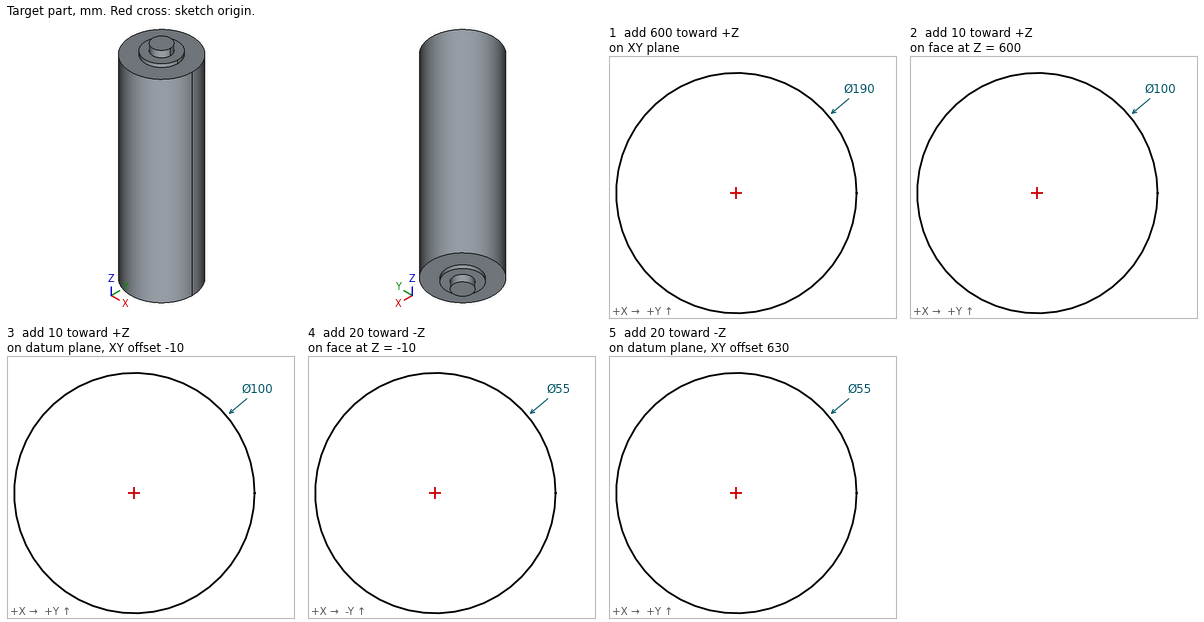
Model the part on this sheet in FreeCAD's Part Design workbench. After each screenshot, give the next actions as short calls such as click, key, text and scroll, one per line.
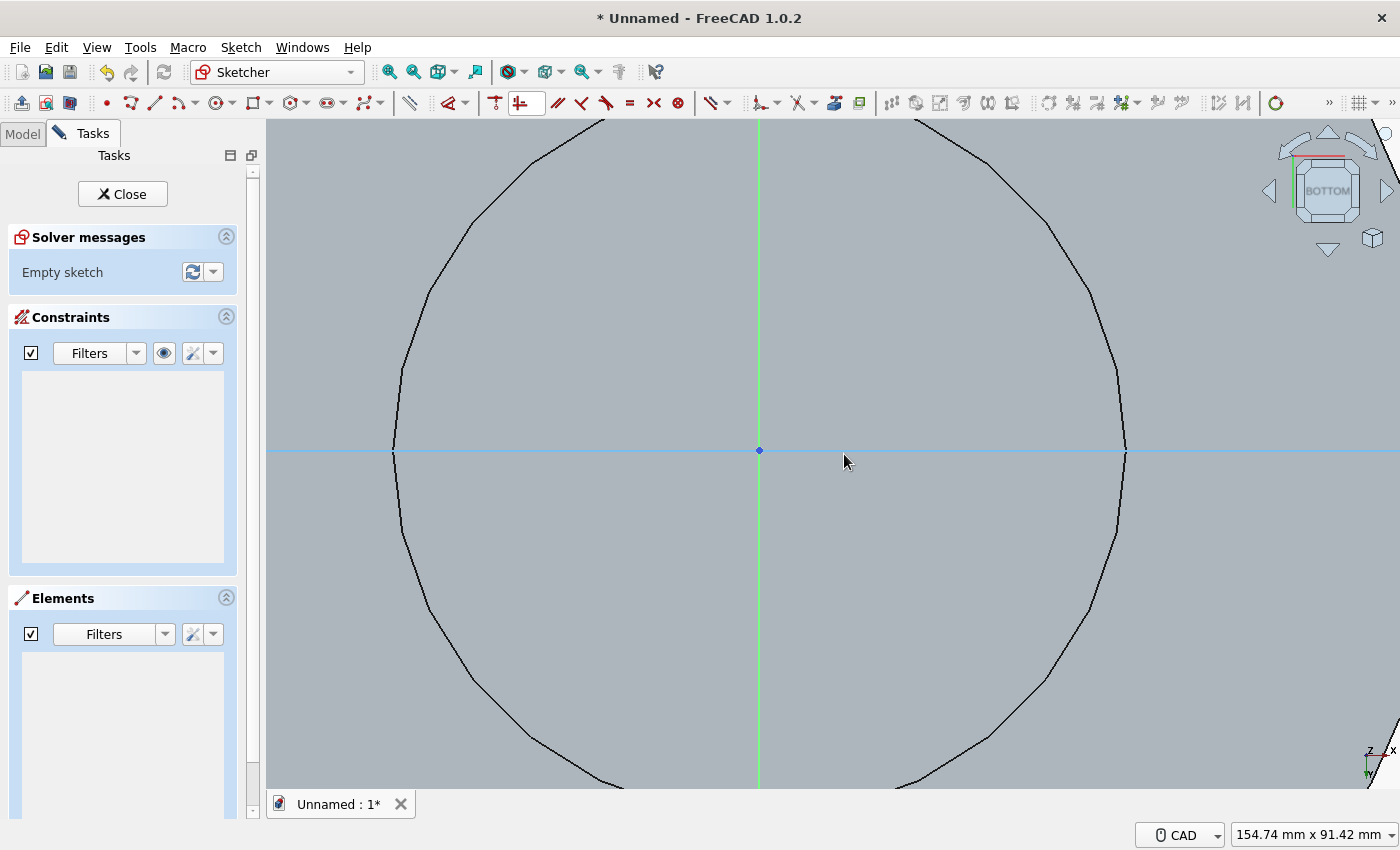
key(g)
key(c)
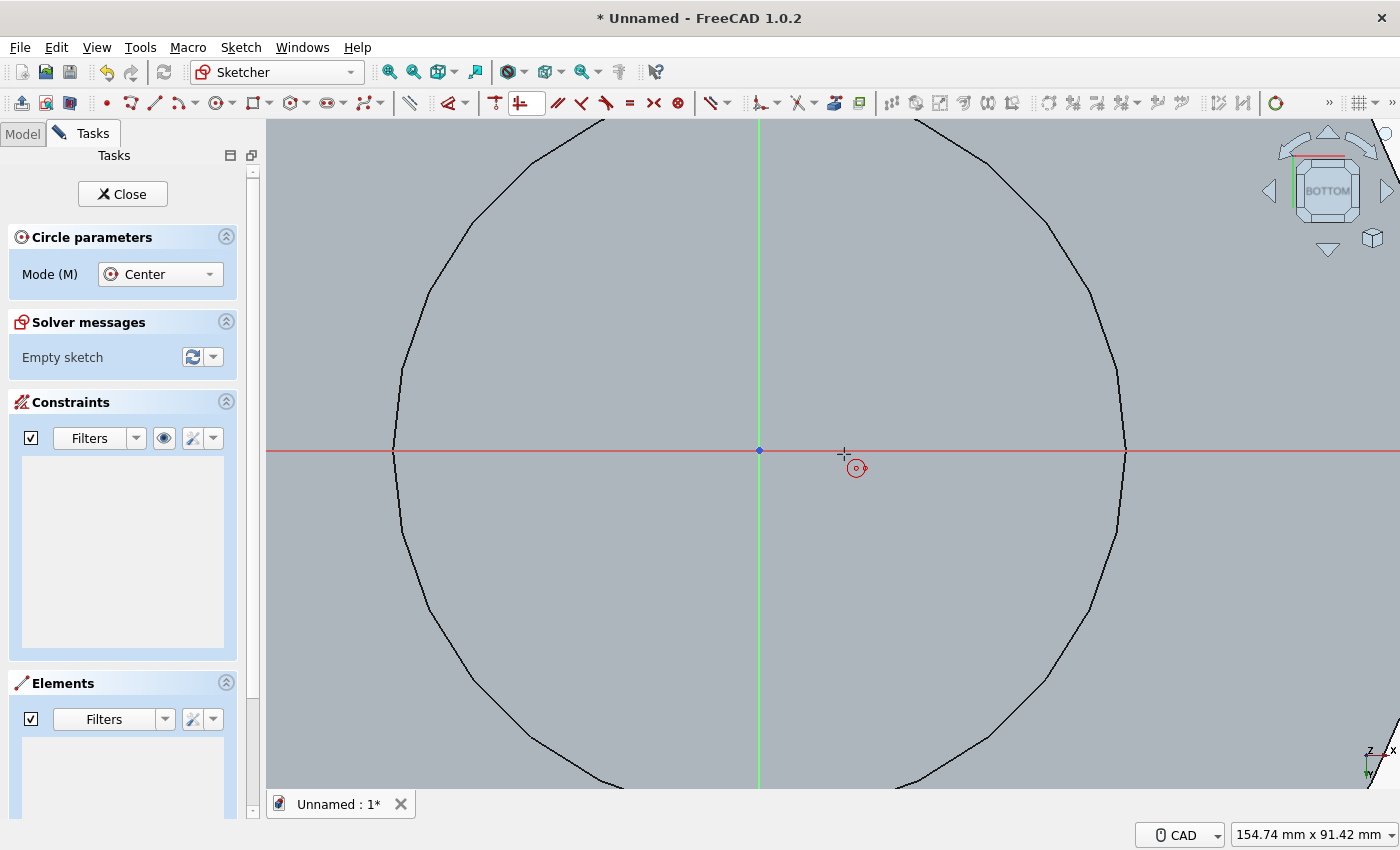
click(759, 451)
click(902, 308)
key(Escape)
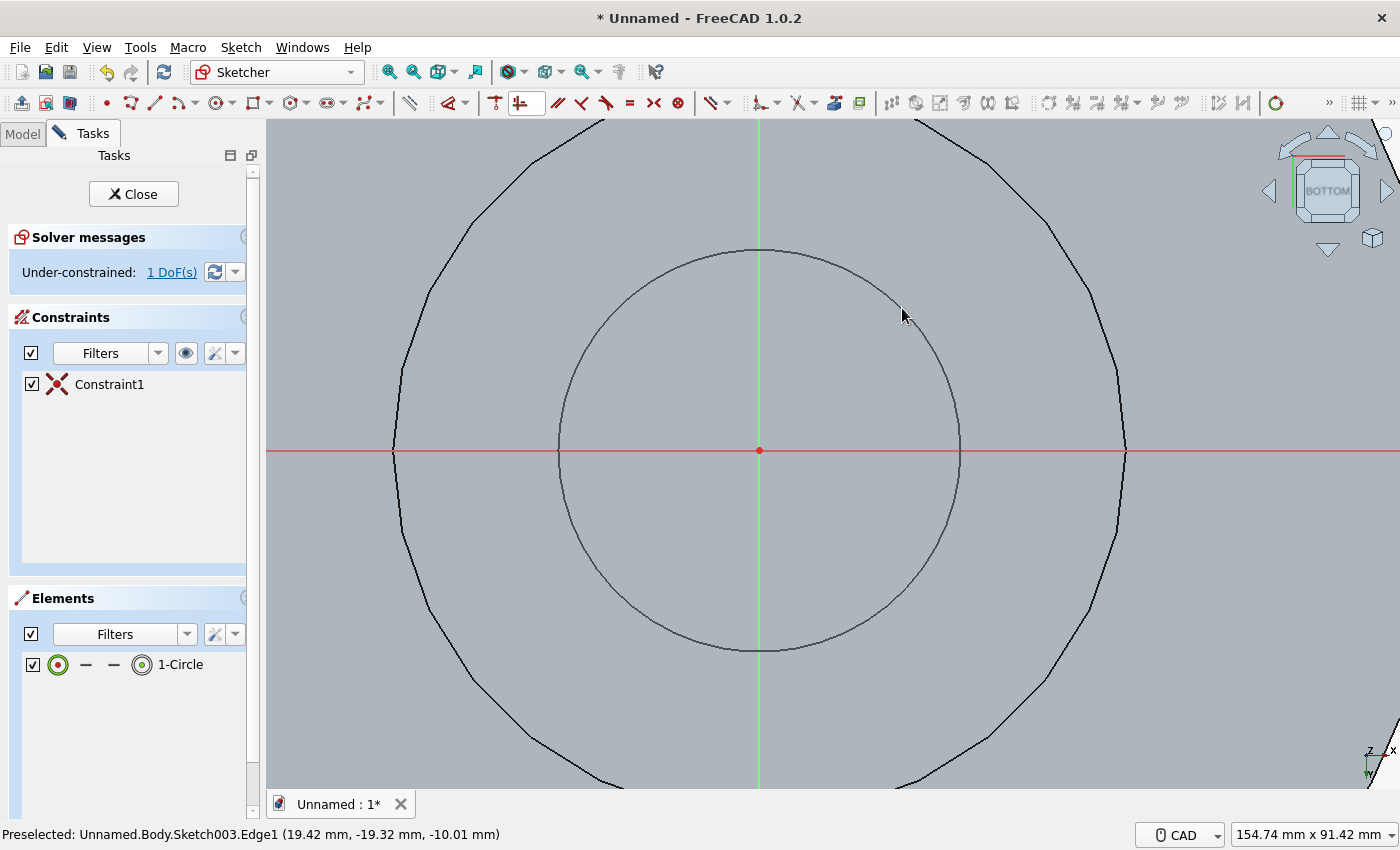
click(448, 104)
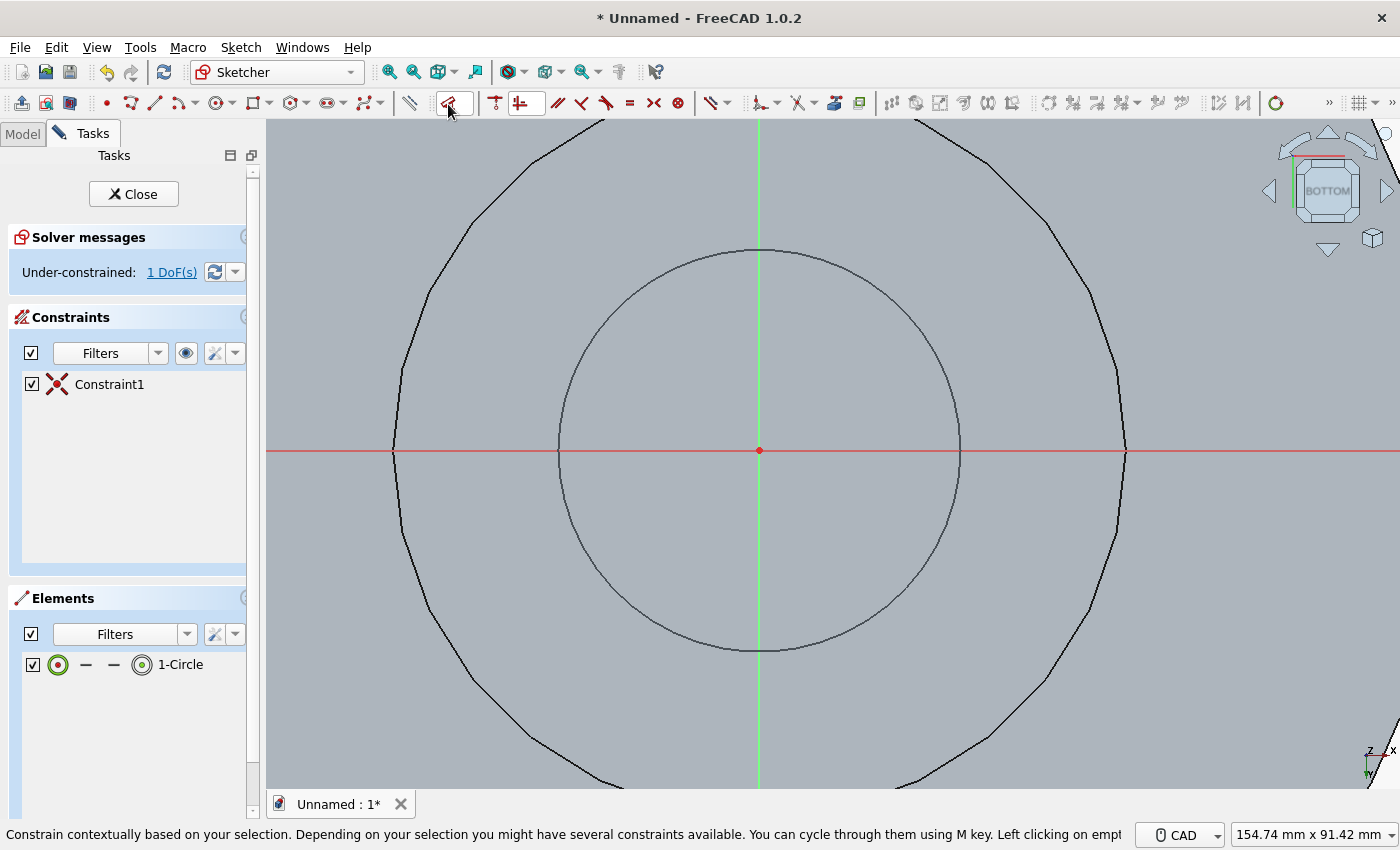
click(901, 308)
click(924, 285)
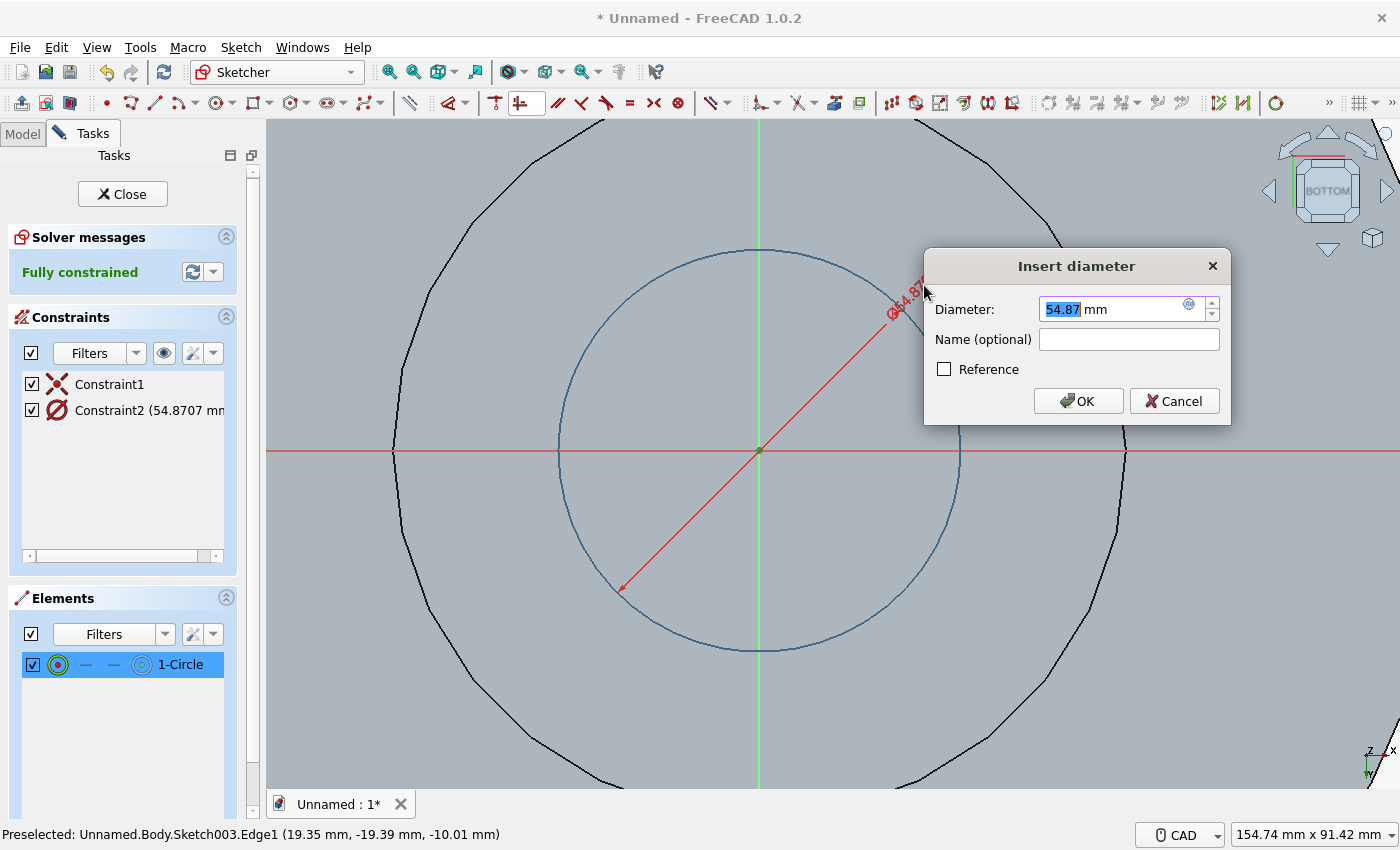
text(55)
key(Return)
key(Escape)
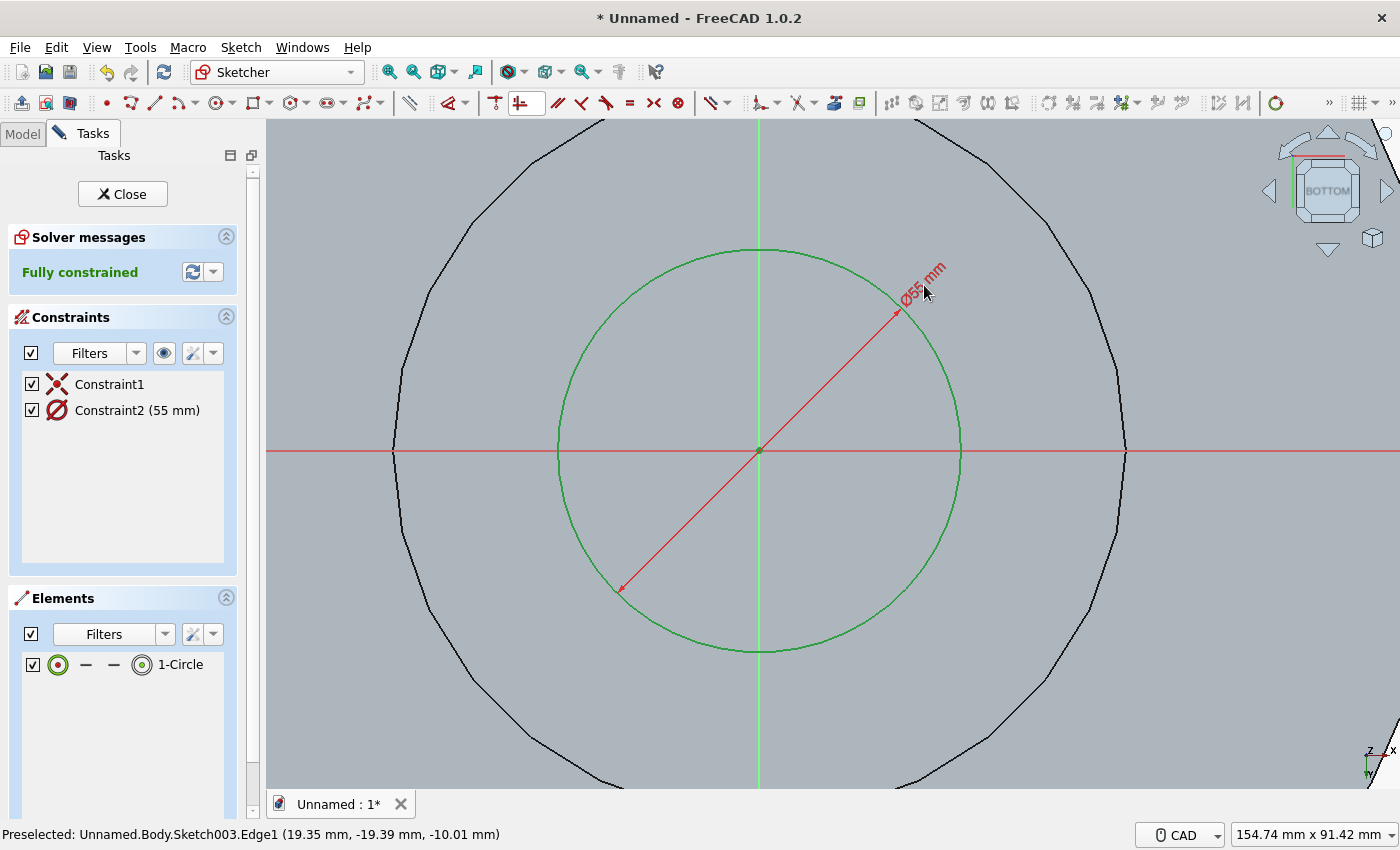
click(123, 194)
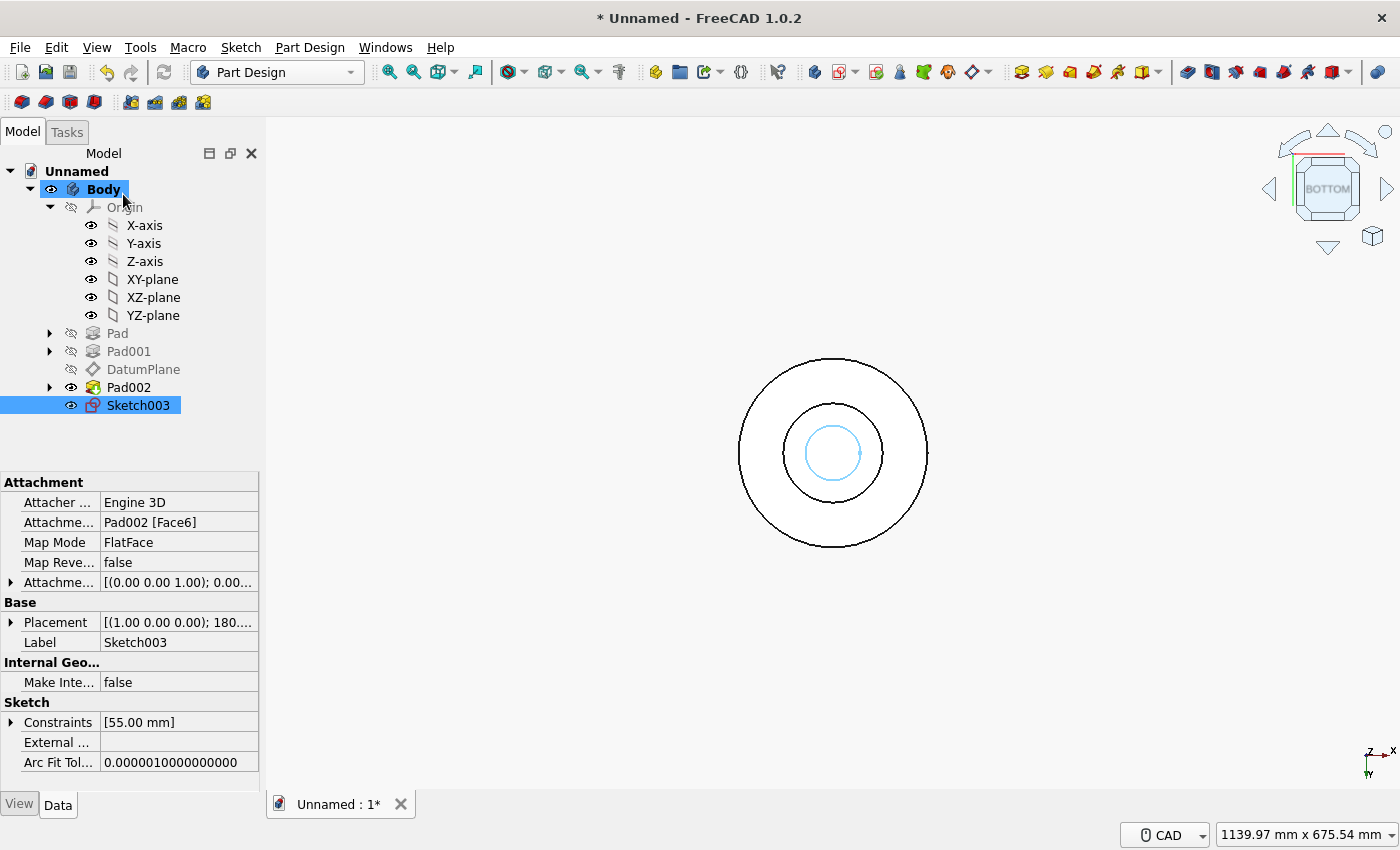
click(1022, 72)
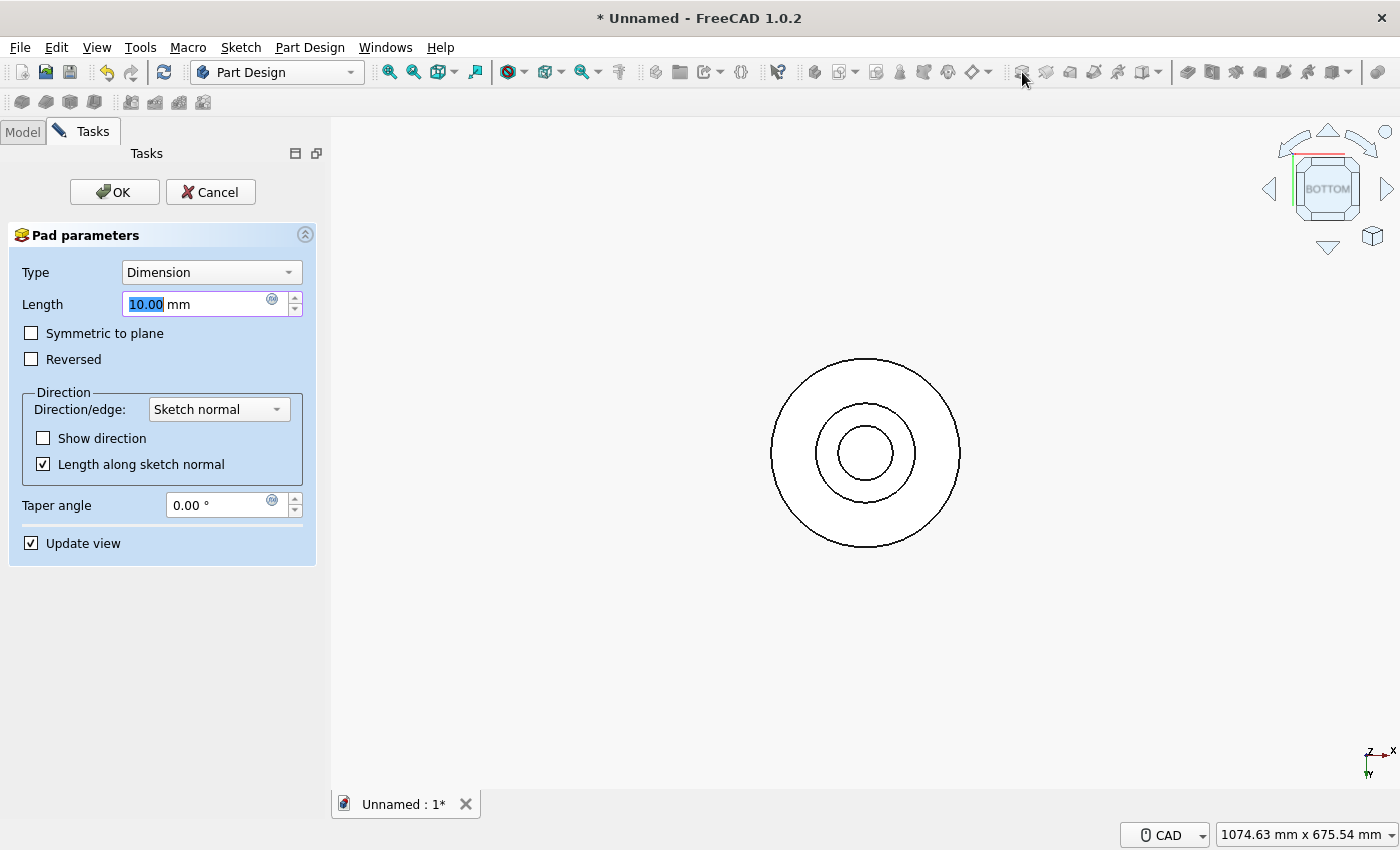
text(20)
key(Tab)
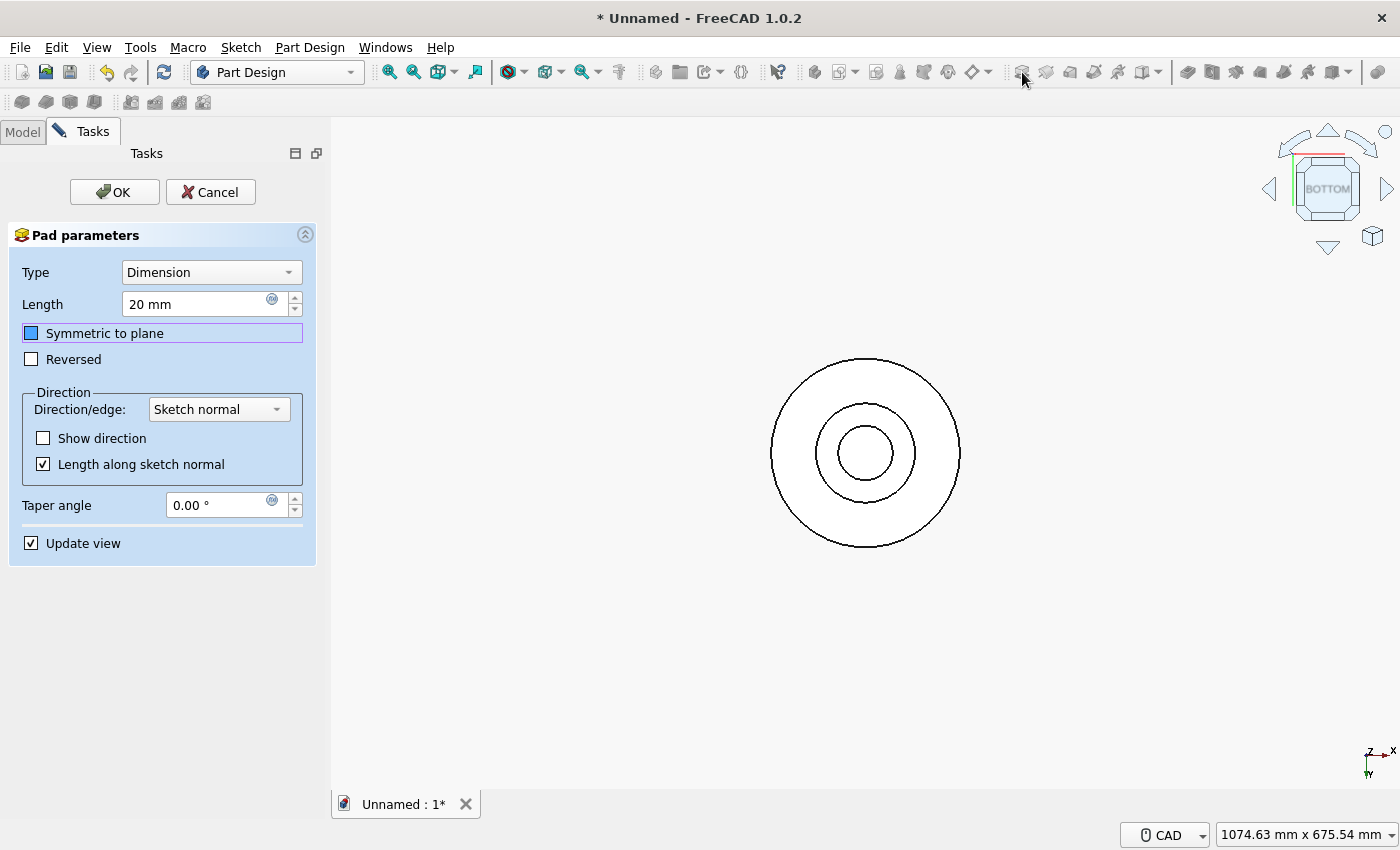
click(115, 192)